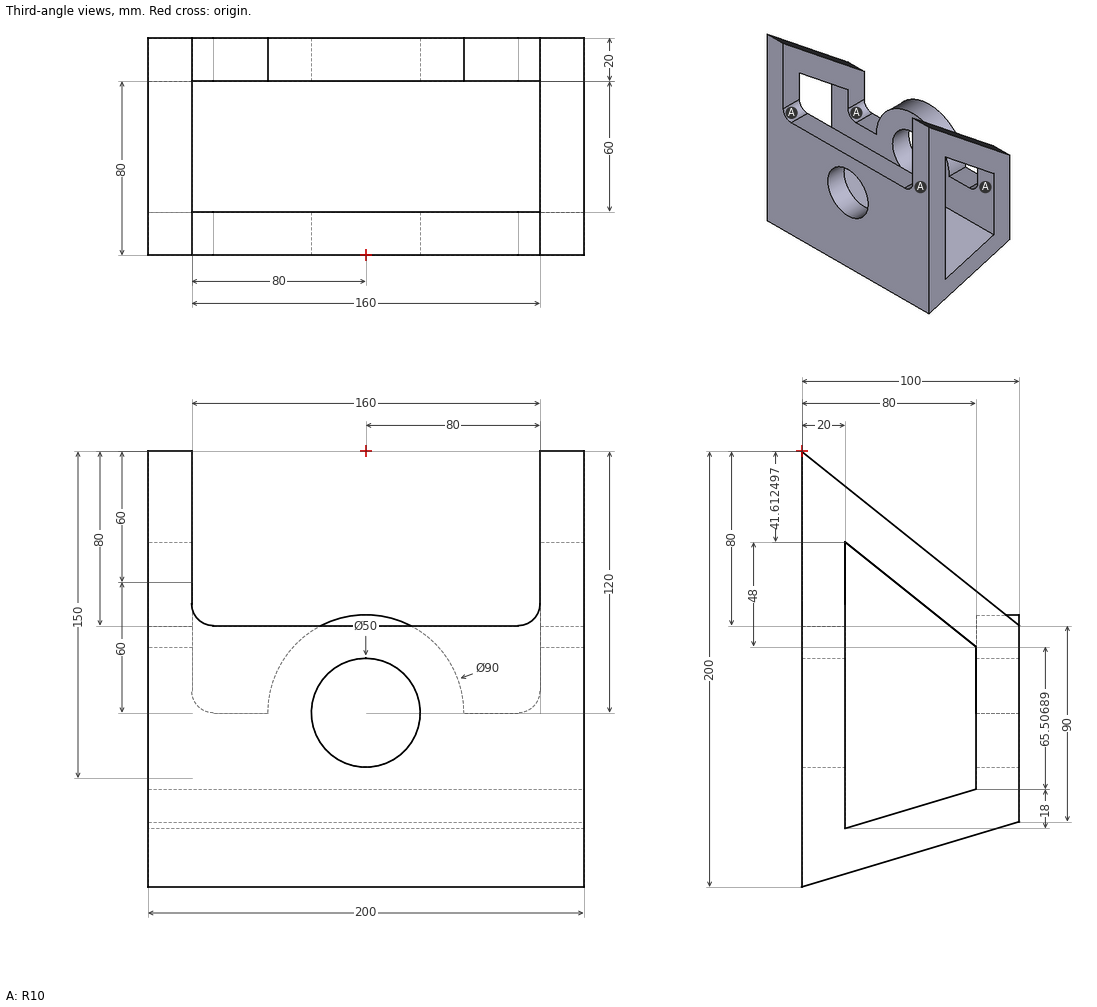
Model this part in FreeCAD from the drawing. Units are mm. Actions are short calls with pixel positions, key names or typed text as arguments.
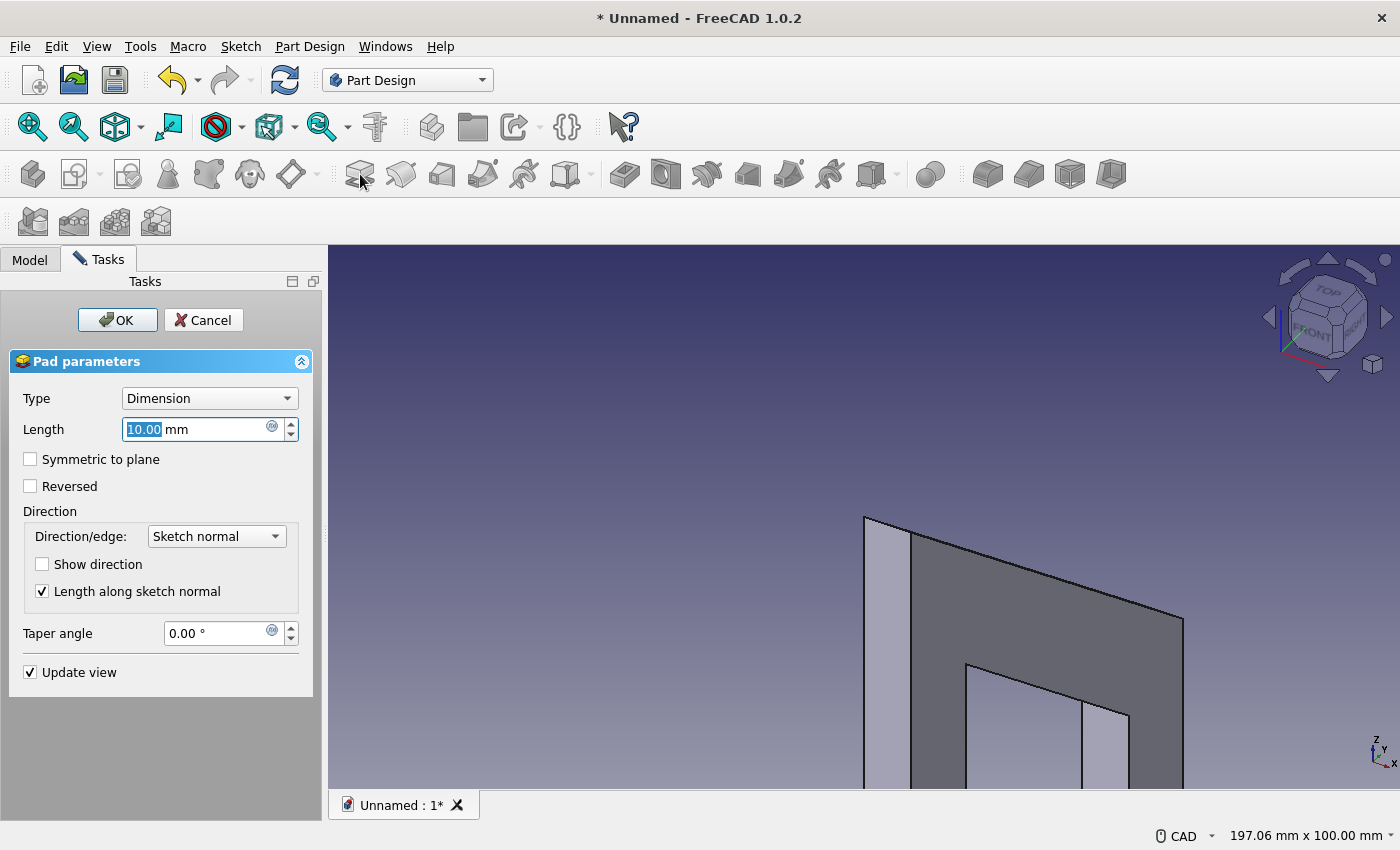
text(200)
key(Tab)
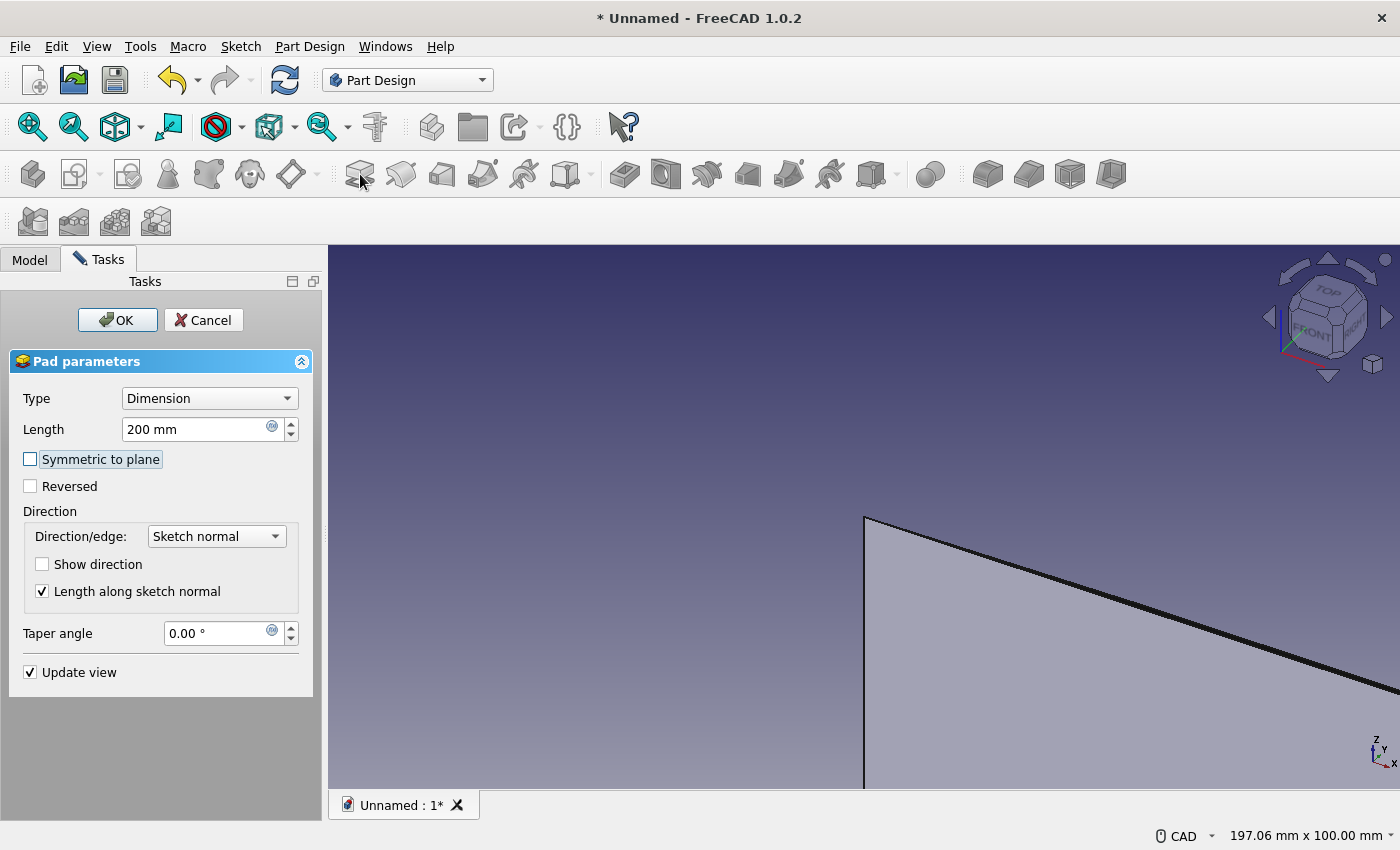
click(31, 459)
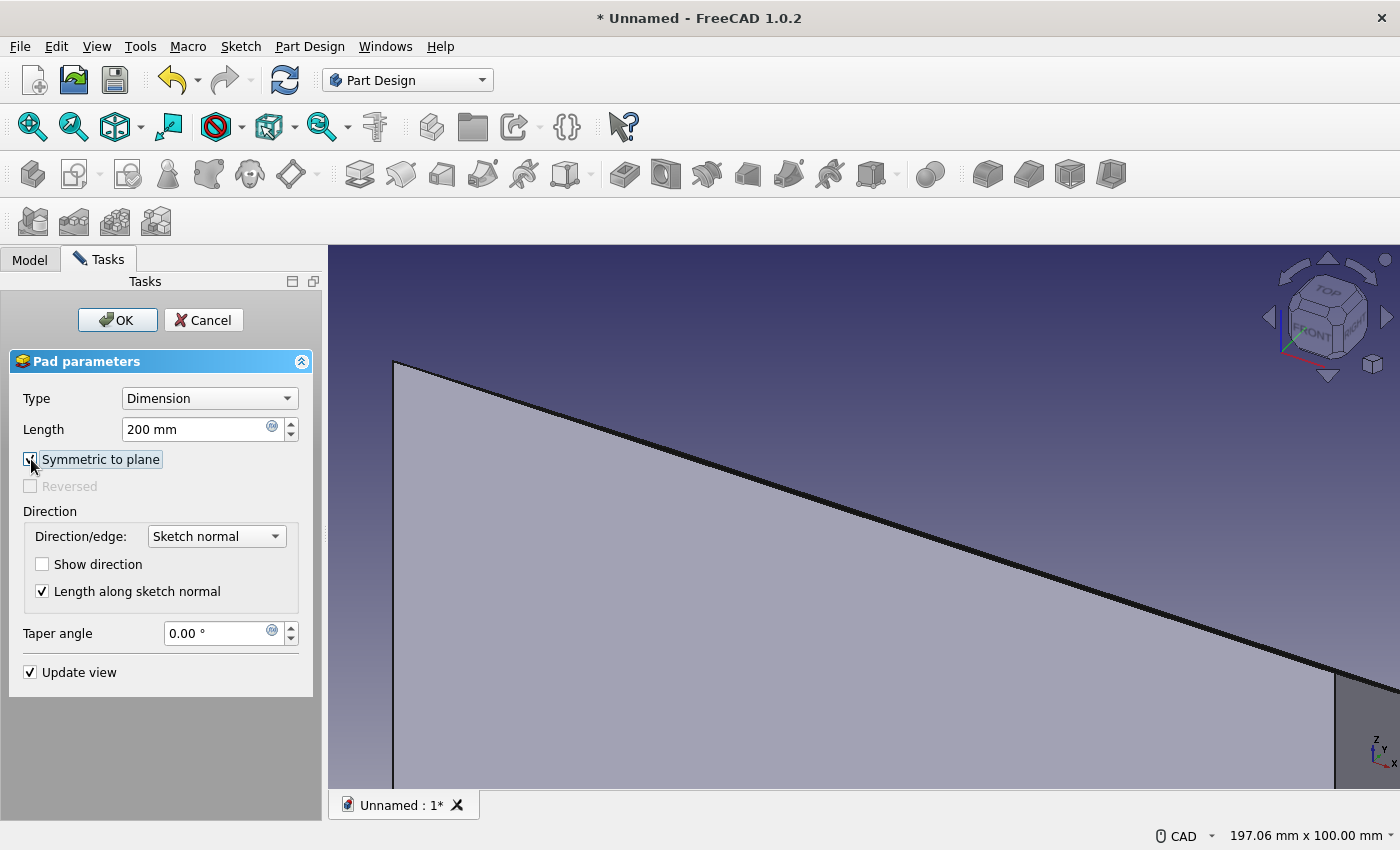
click(118, 320)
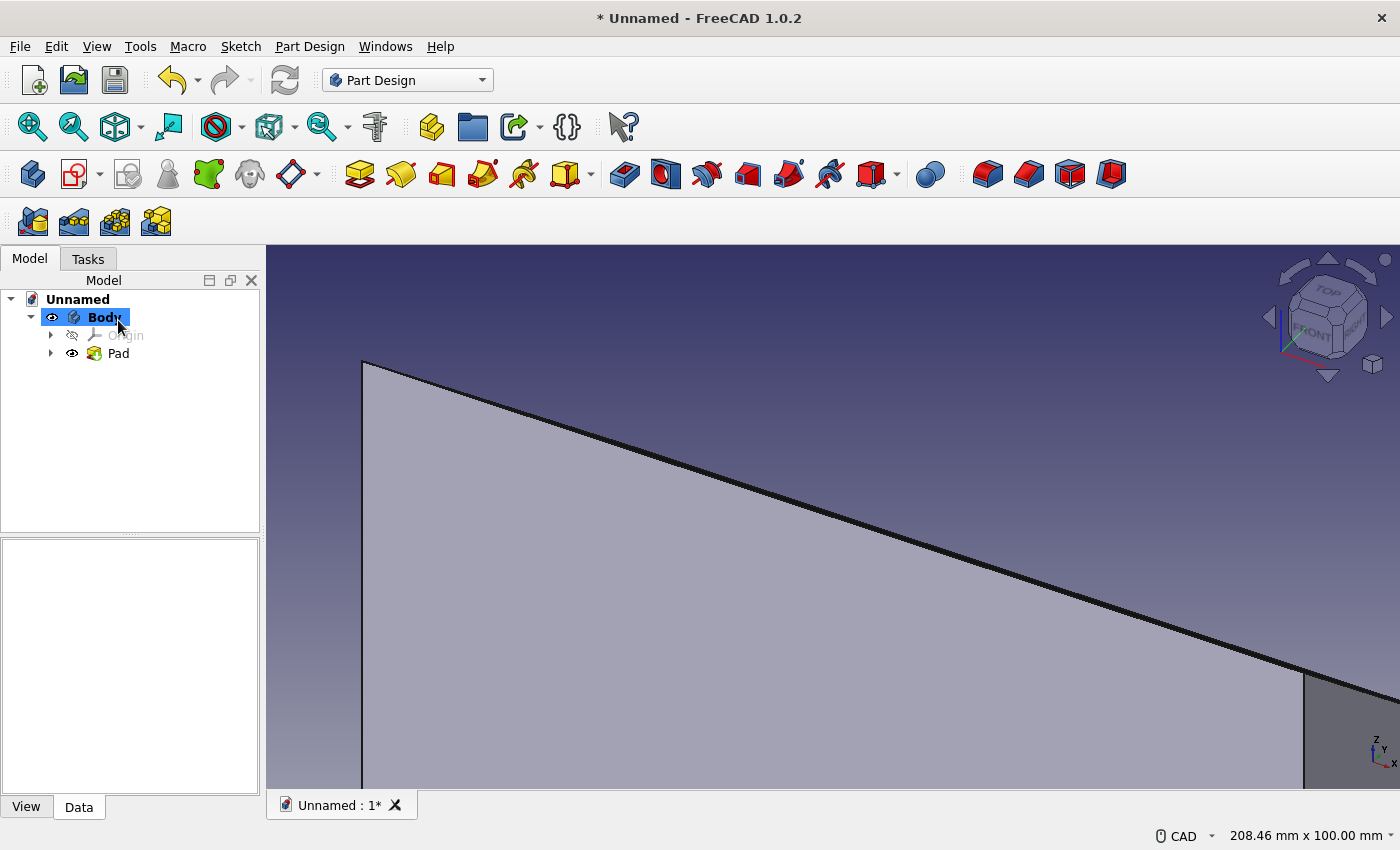
key(v)
key(f)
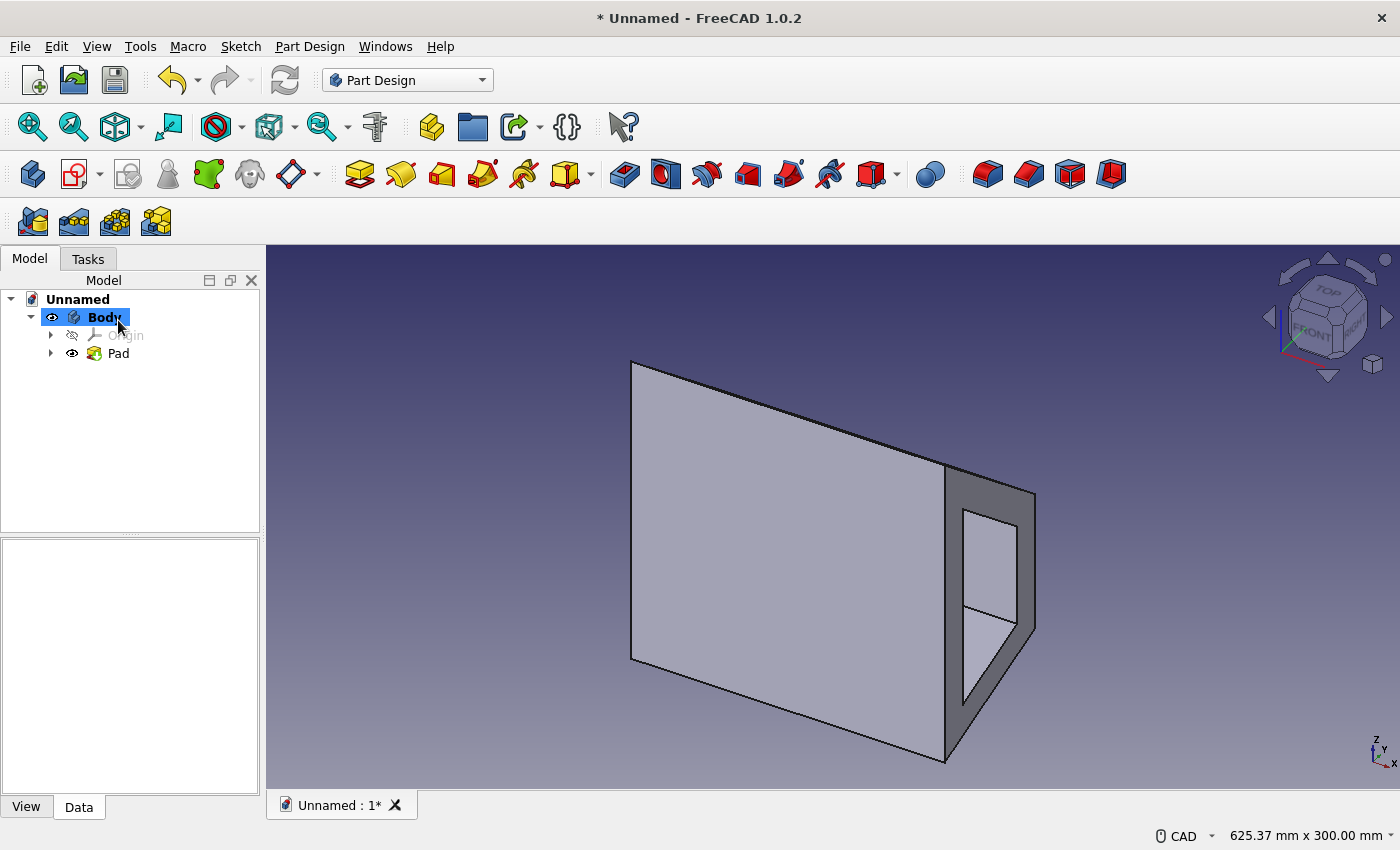
click(74, 174)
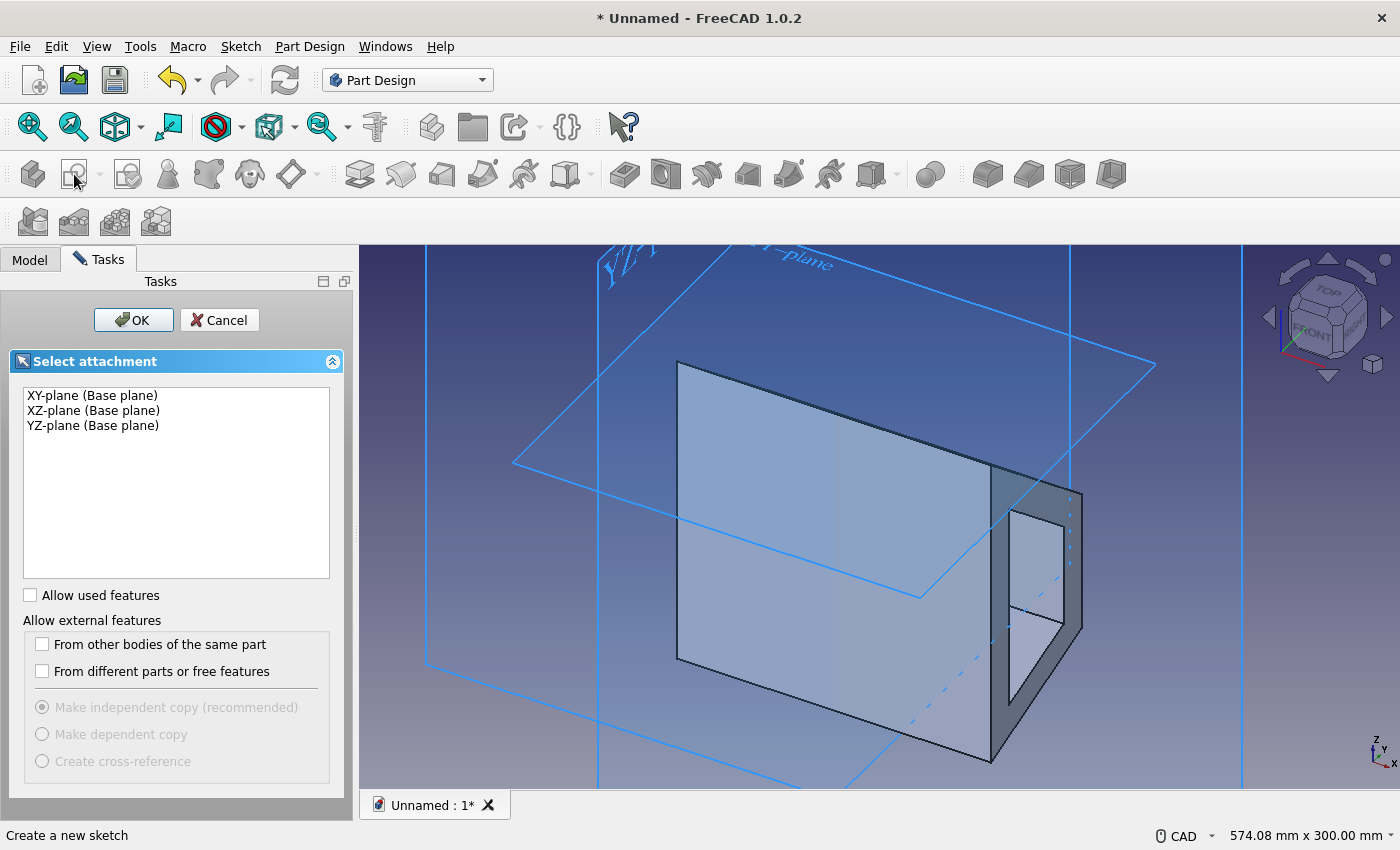
click(84, 396)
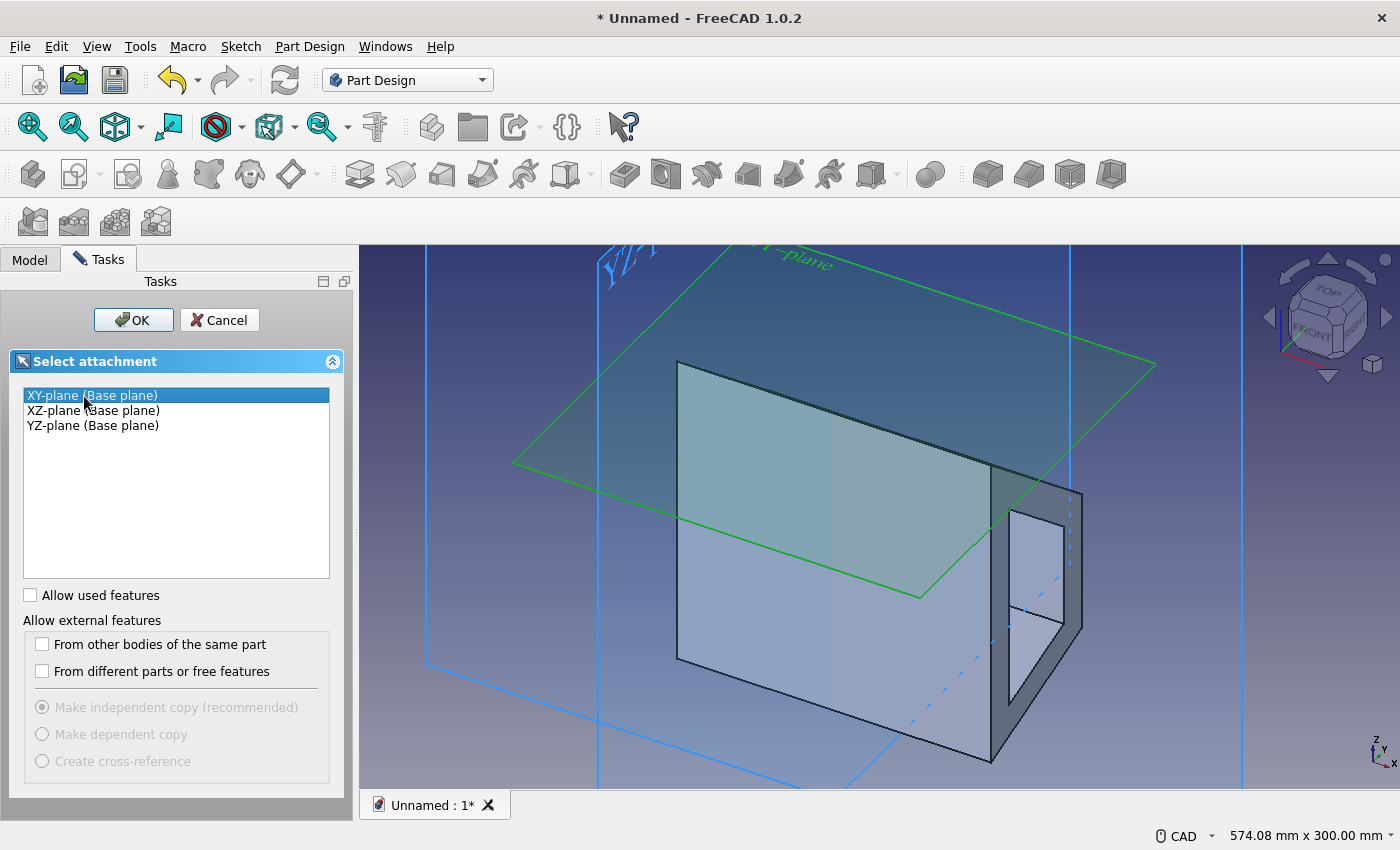
click(134, 320)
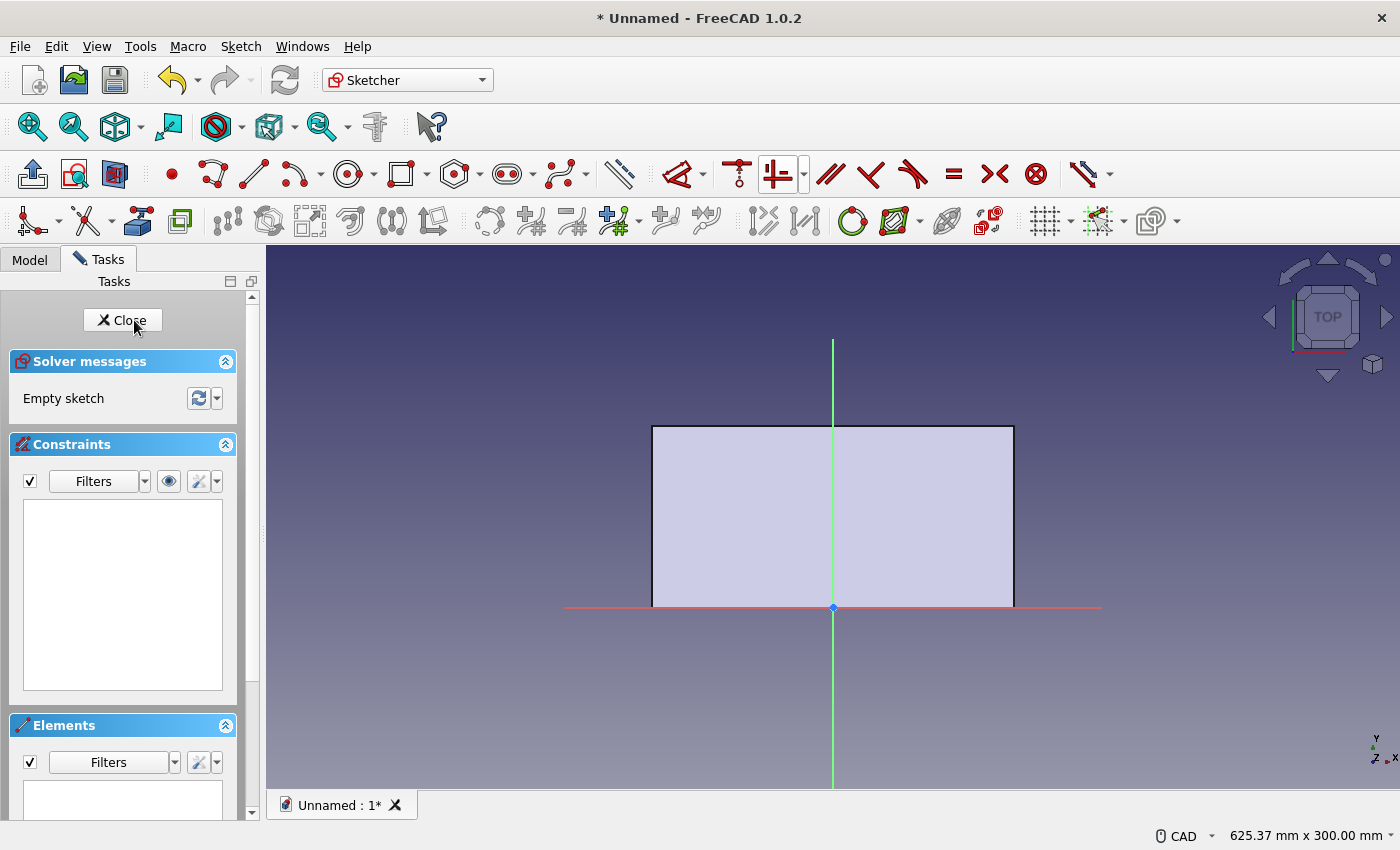
scroll(889, 550, up, 4)